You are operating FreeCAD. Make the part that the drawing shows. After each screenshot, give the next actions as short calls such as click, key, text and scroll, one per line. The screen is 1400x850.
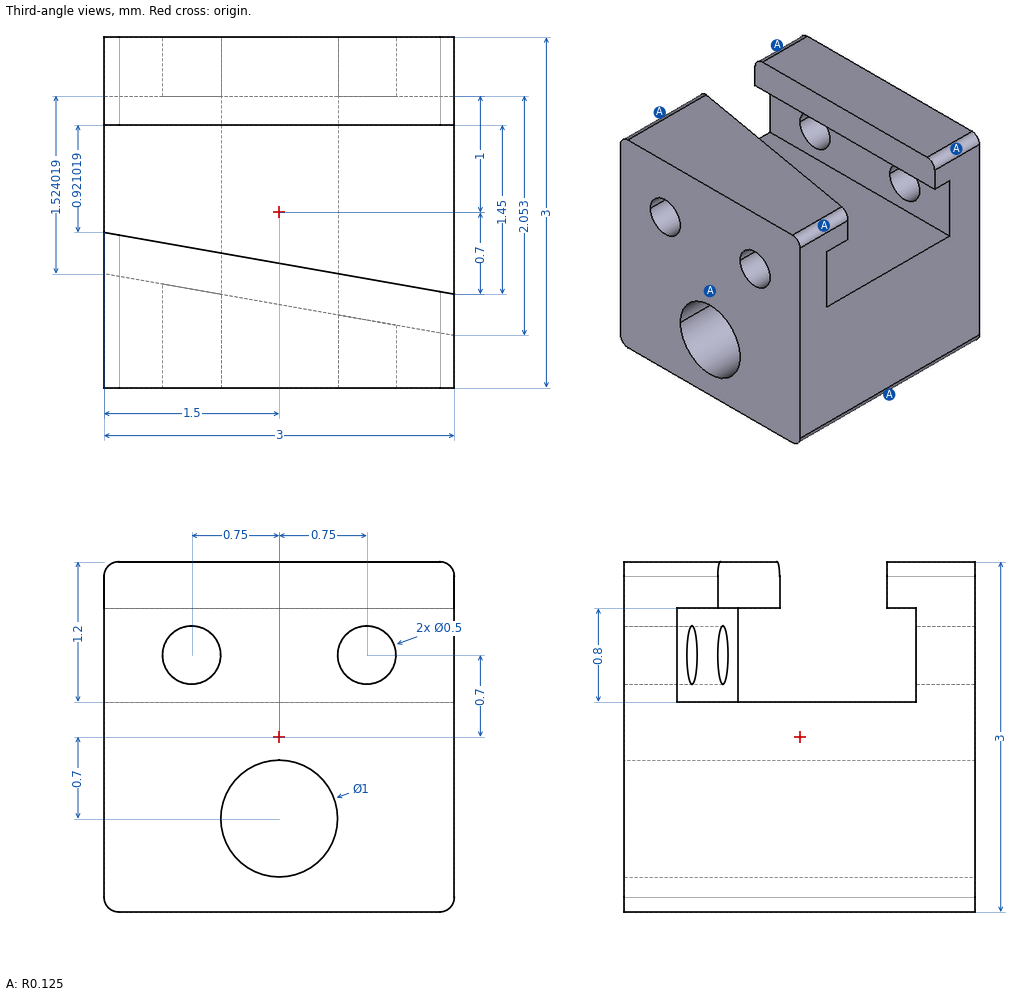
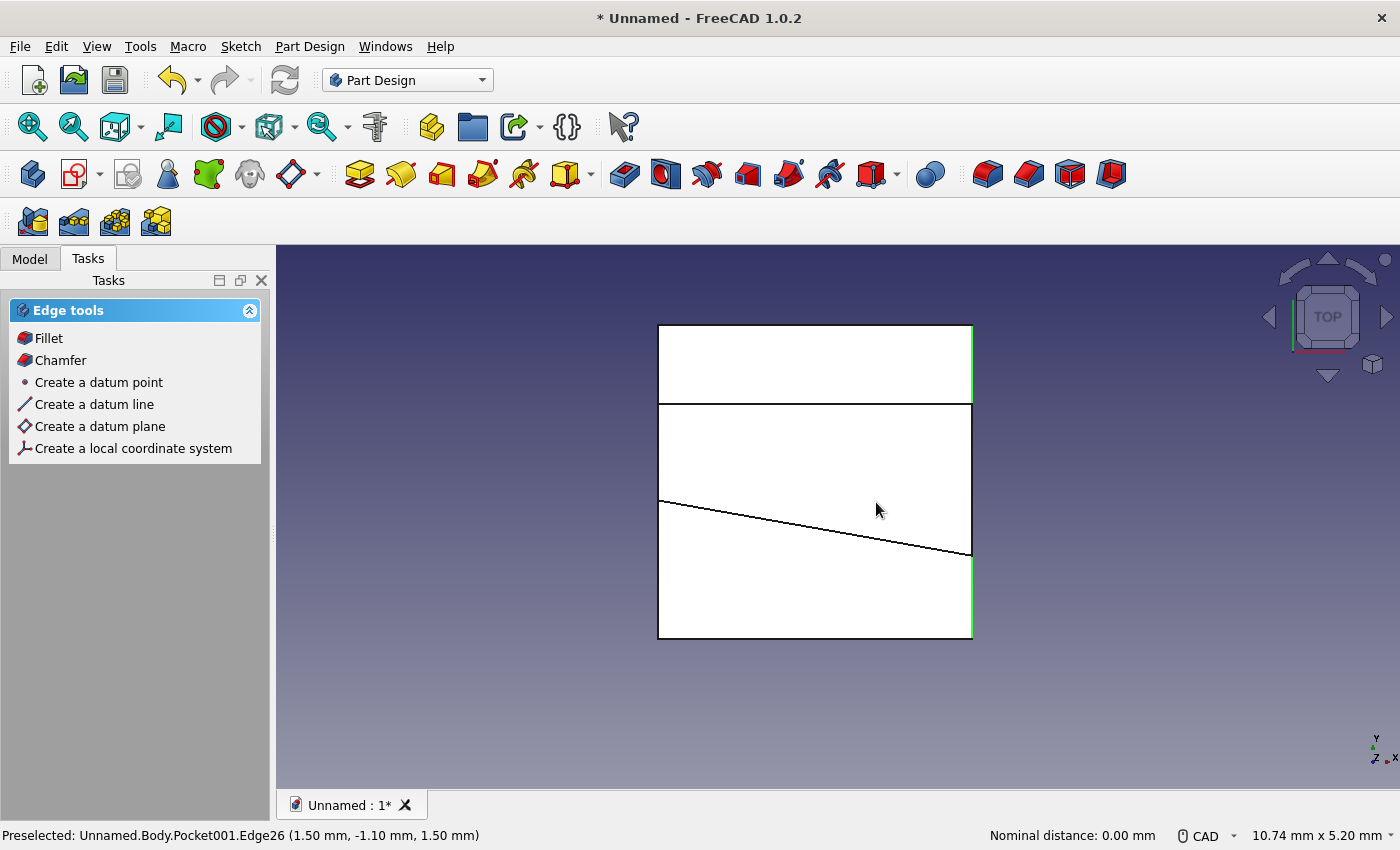
click(658, 364, ctrl)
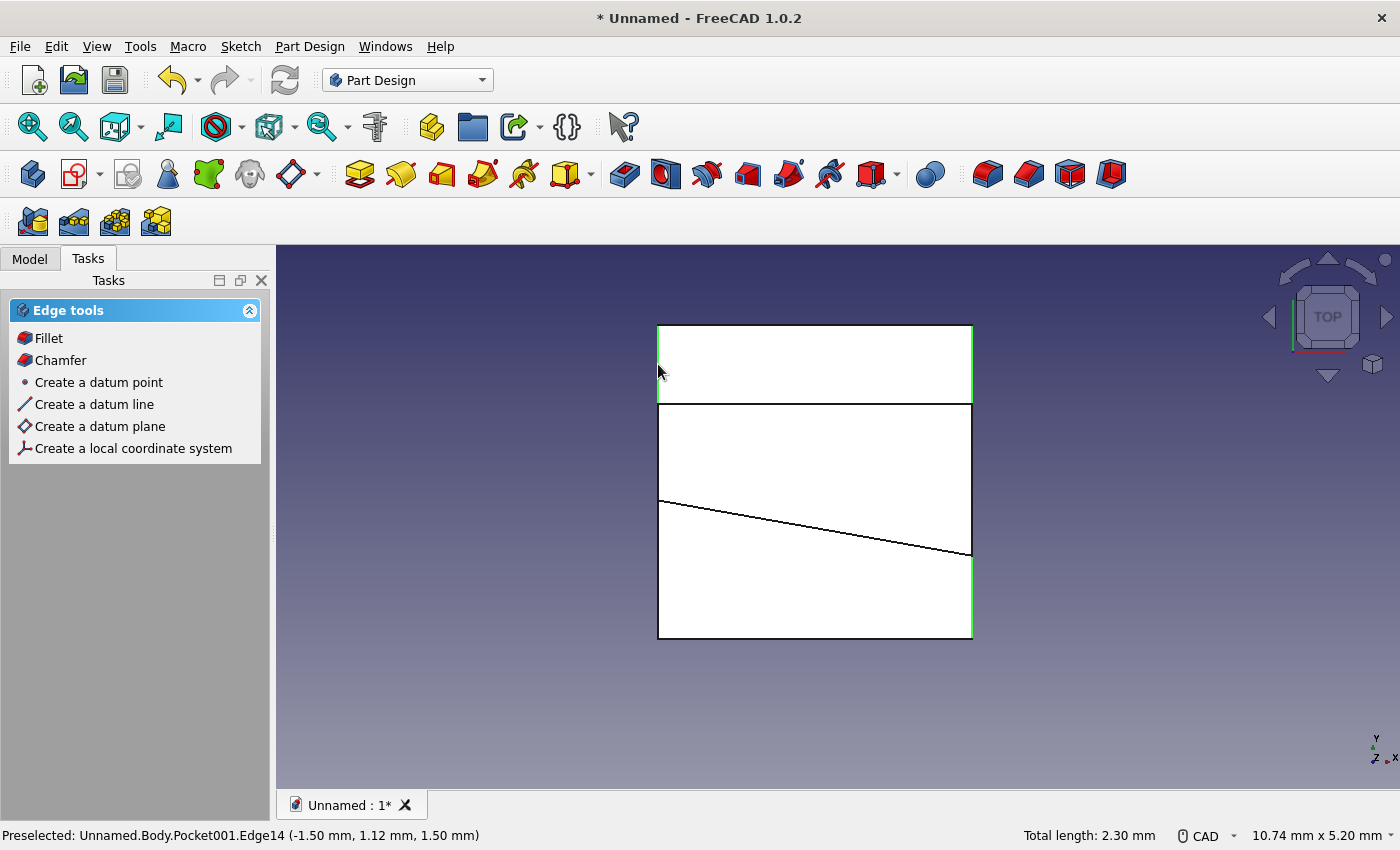
click(658, 569, ctrl)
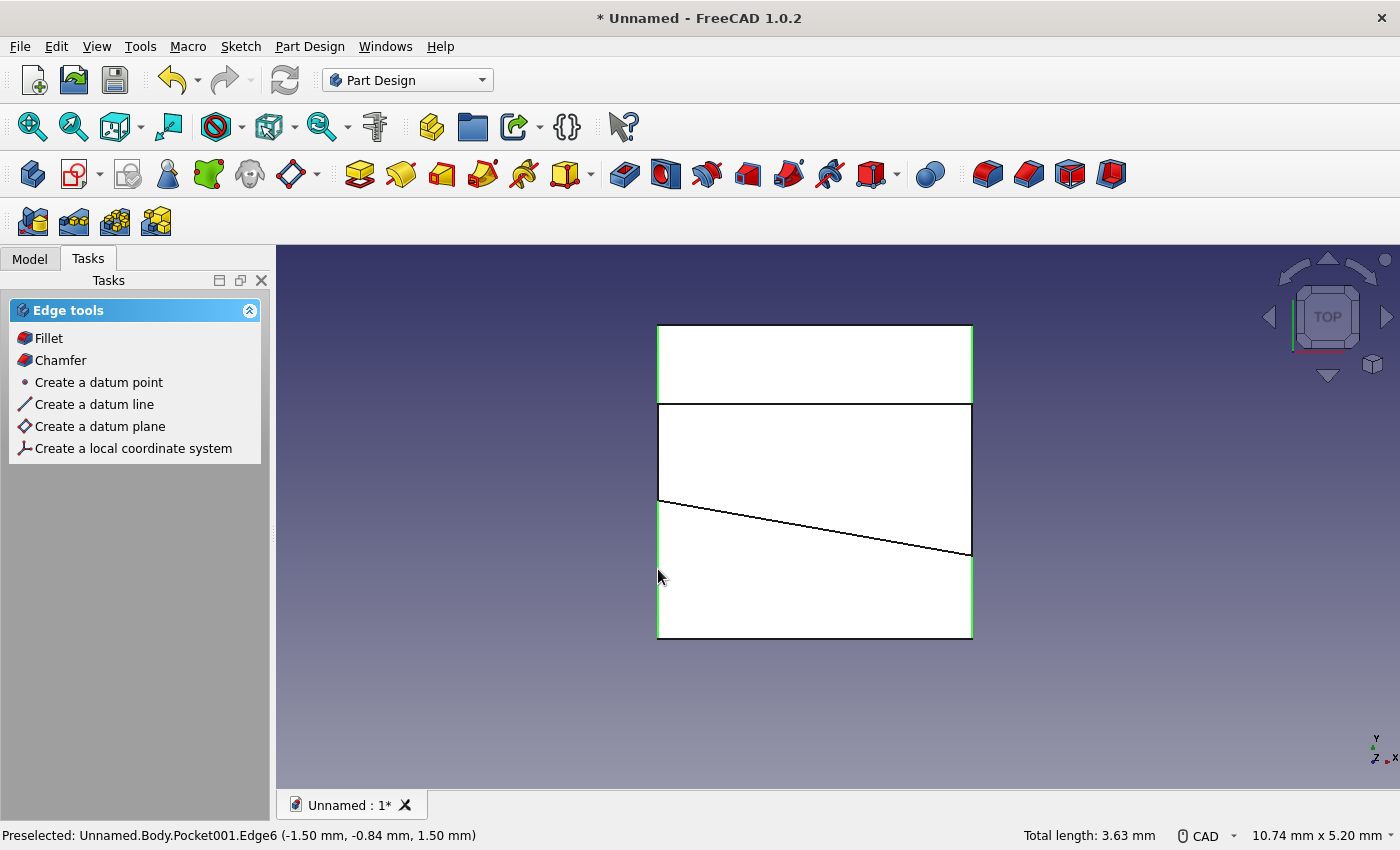
key(0)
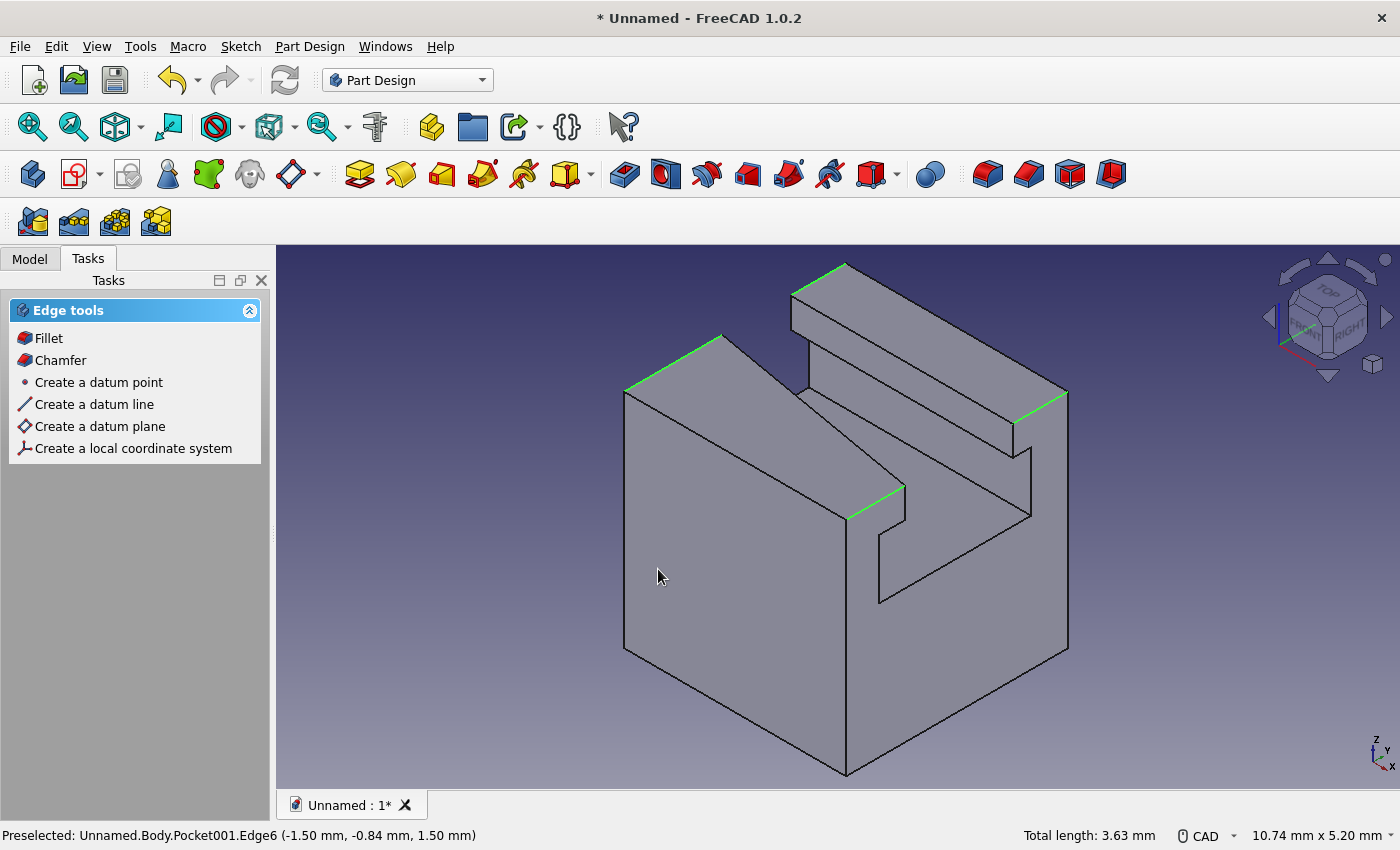
key(1)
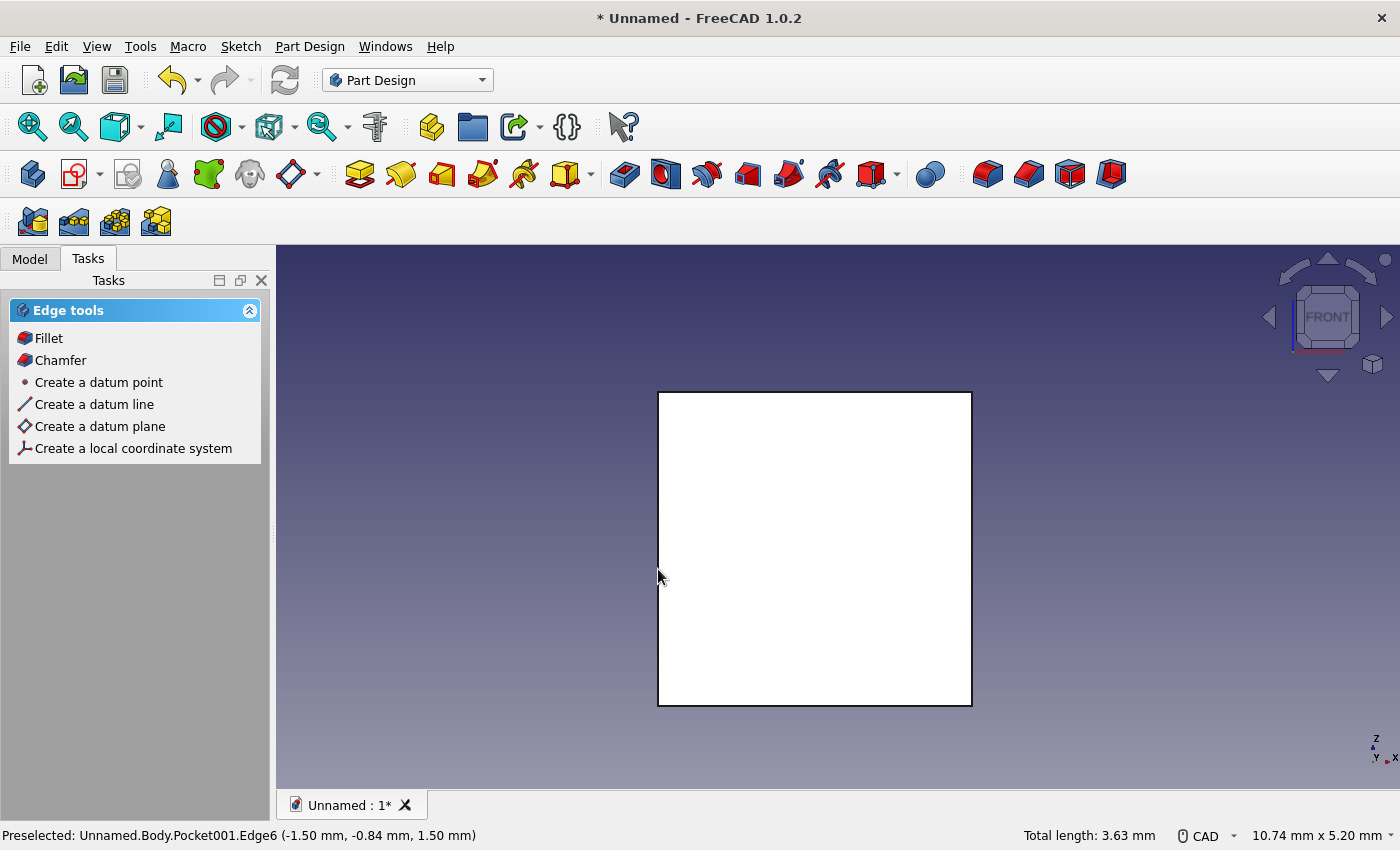
key(3)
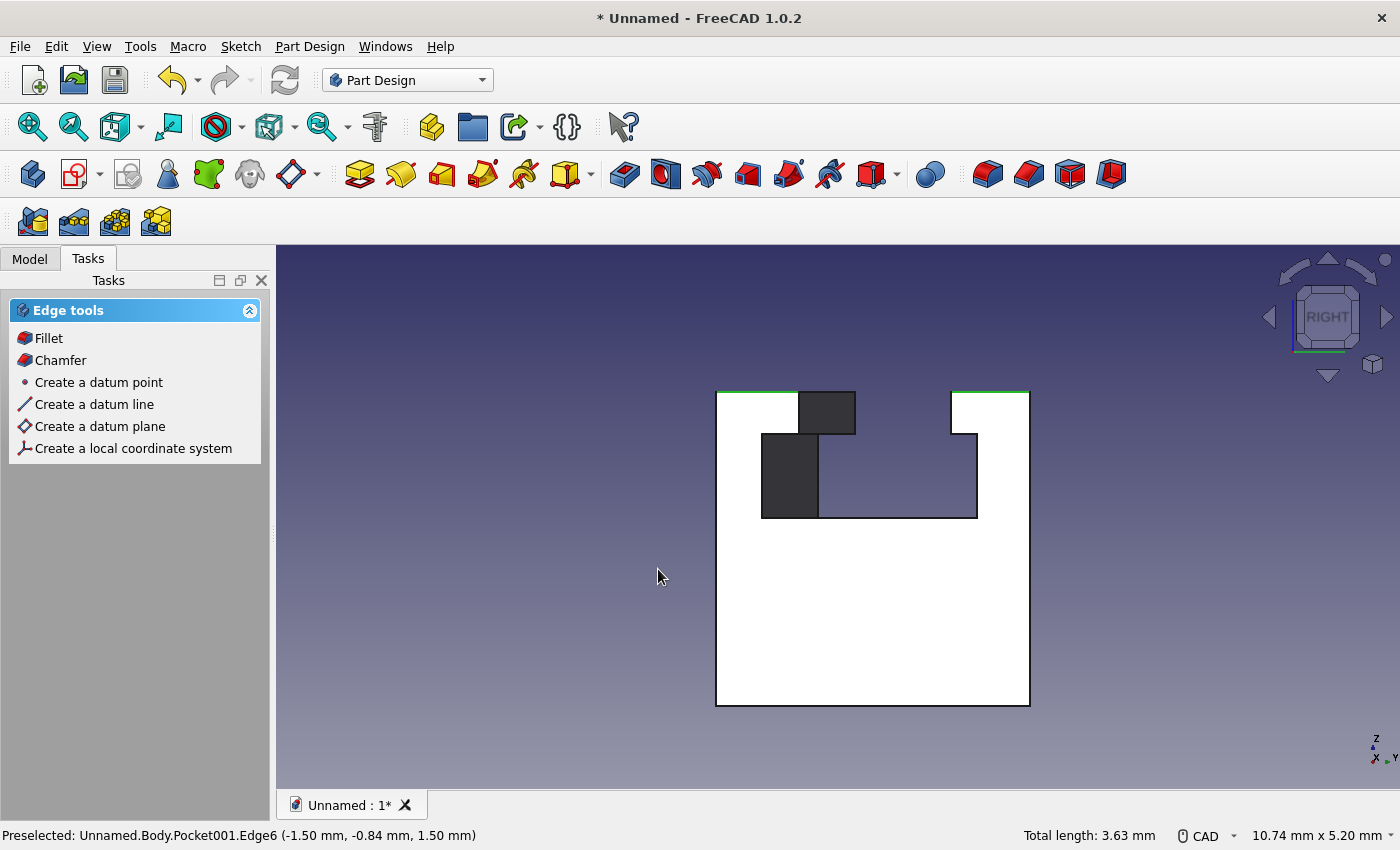
click(873, 705, ctrl)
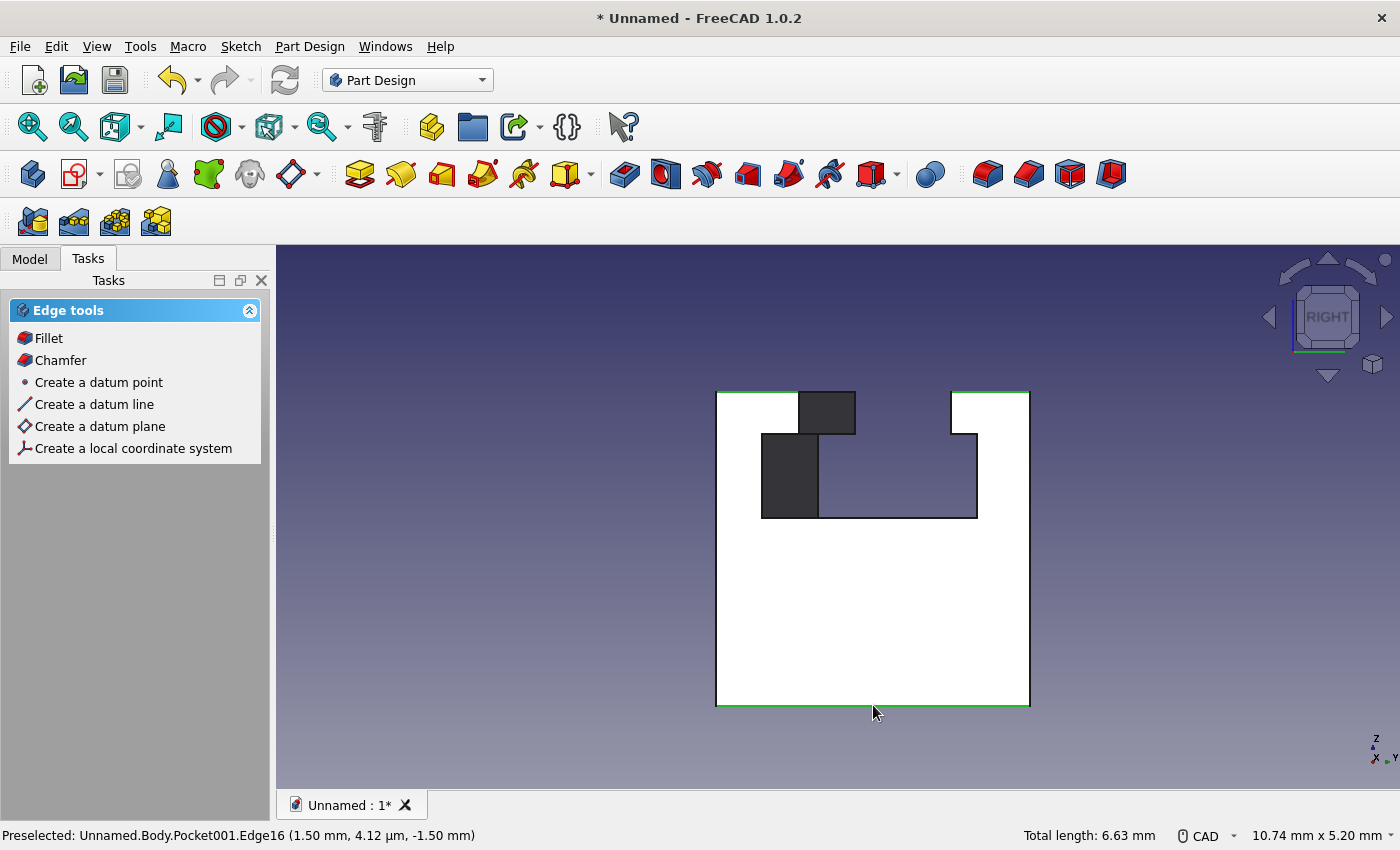
key(5)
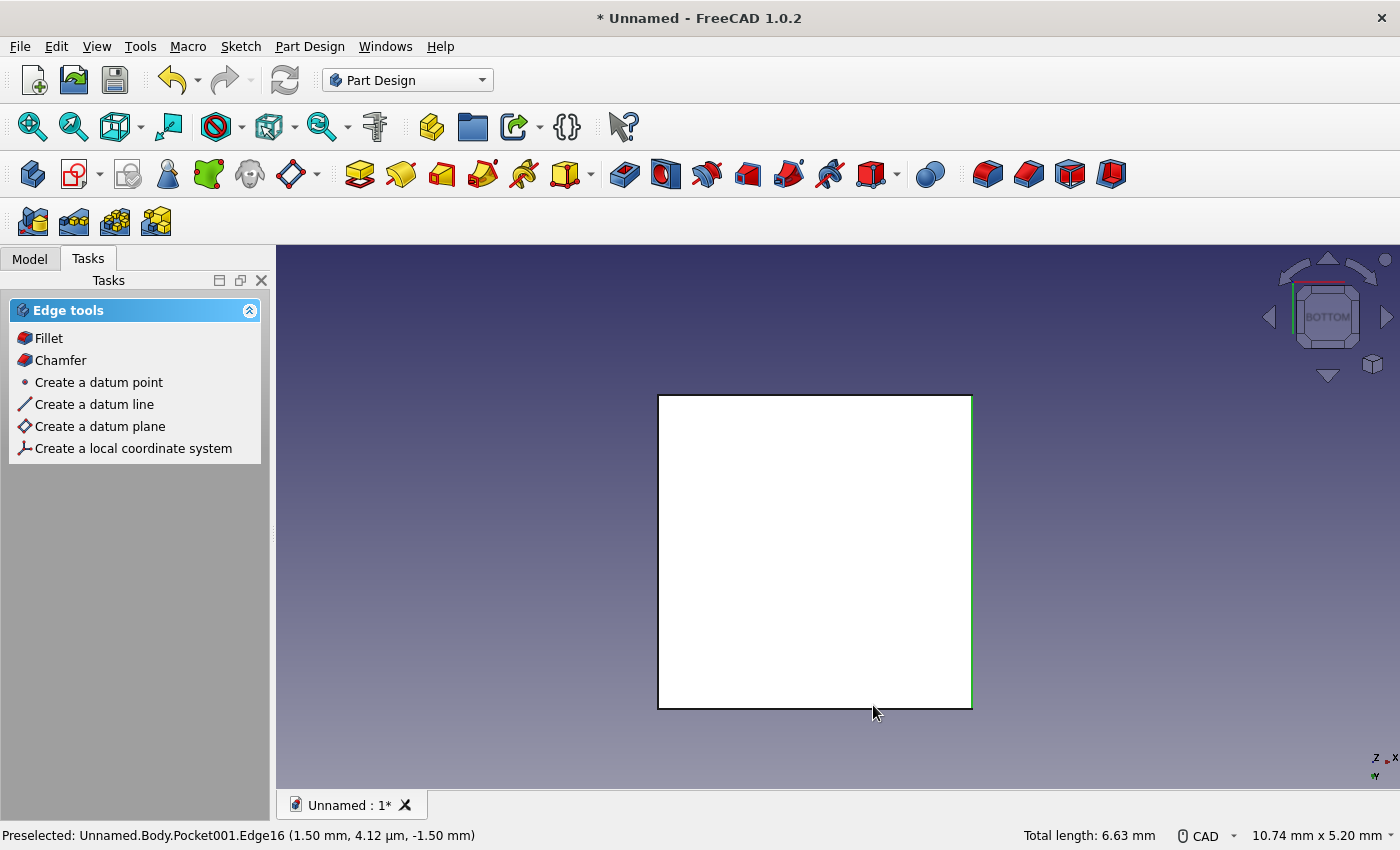
click(658, 551, ctrl)